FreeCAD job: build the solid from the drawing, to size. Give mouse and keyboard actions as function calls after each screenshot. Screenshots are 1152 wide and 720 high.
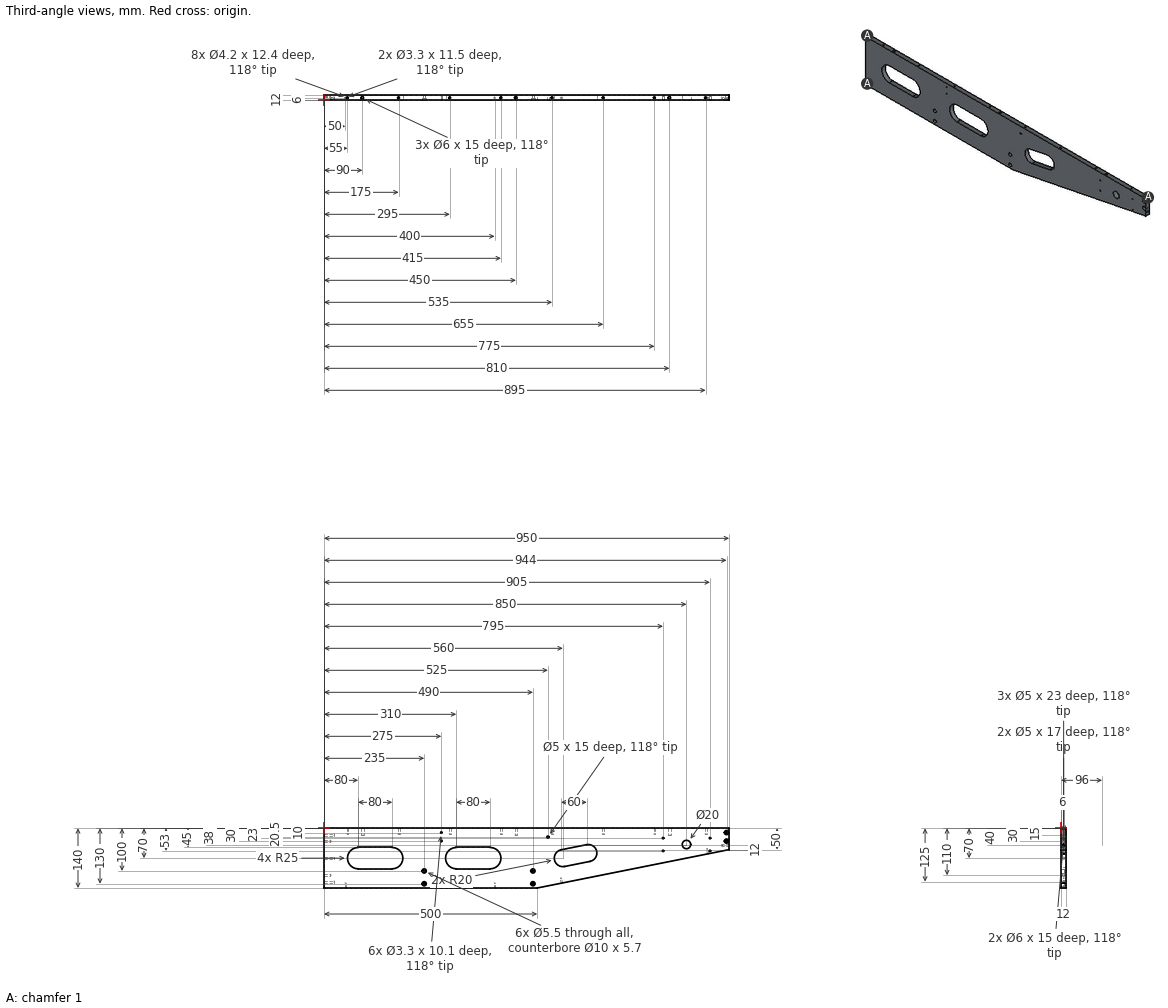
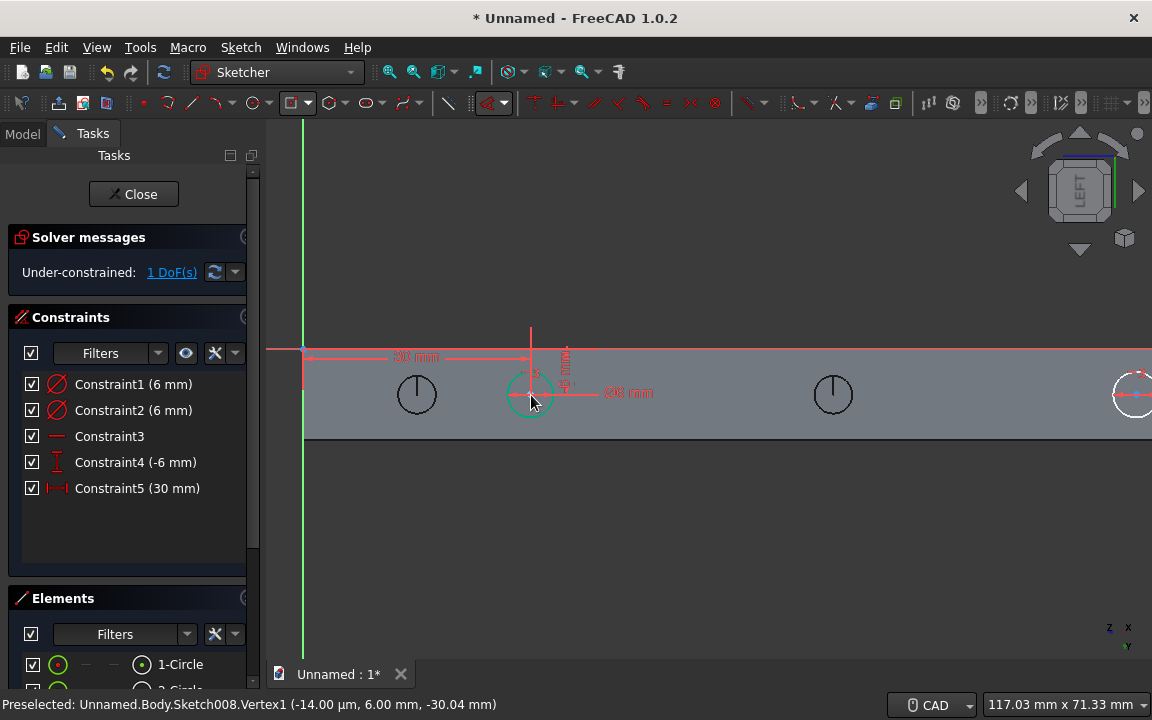
scroll(530, 396, down, 3)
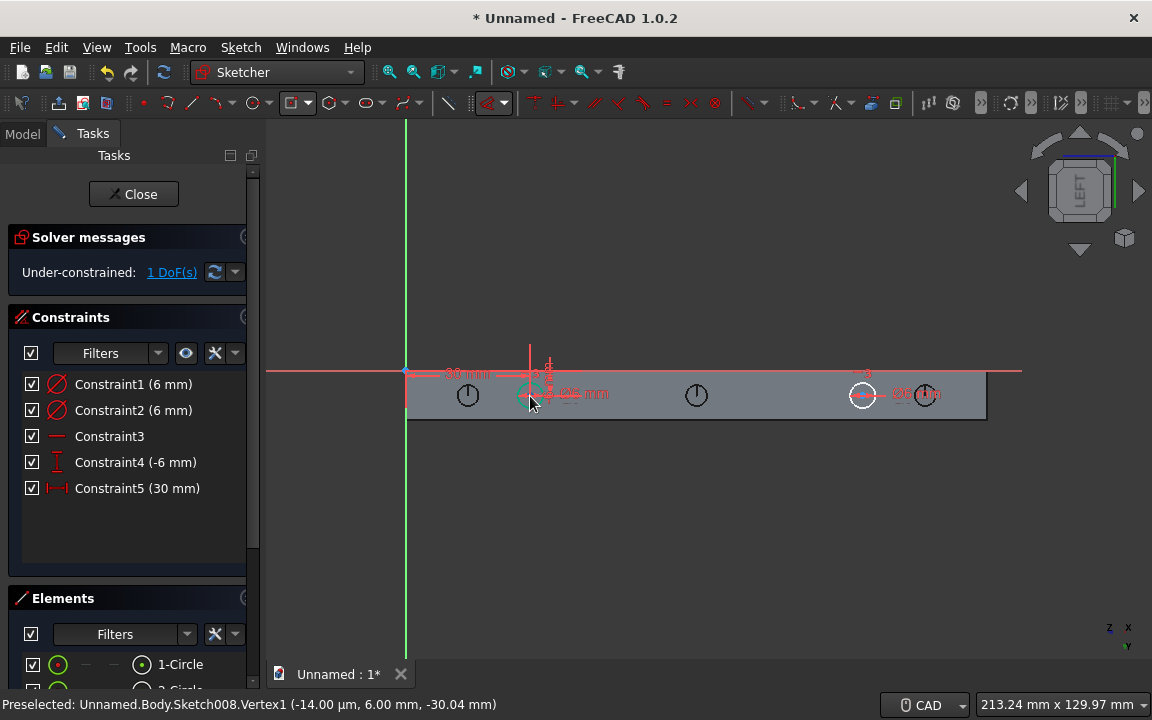
click(863, 396)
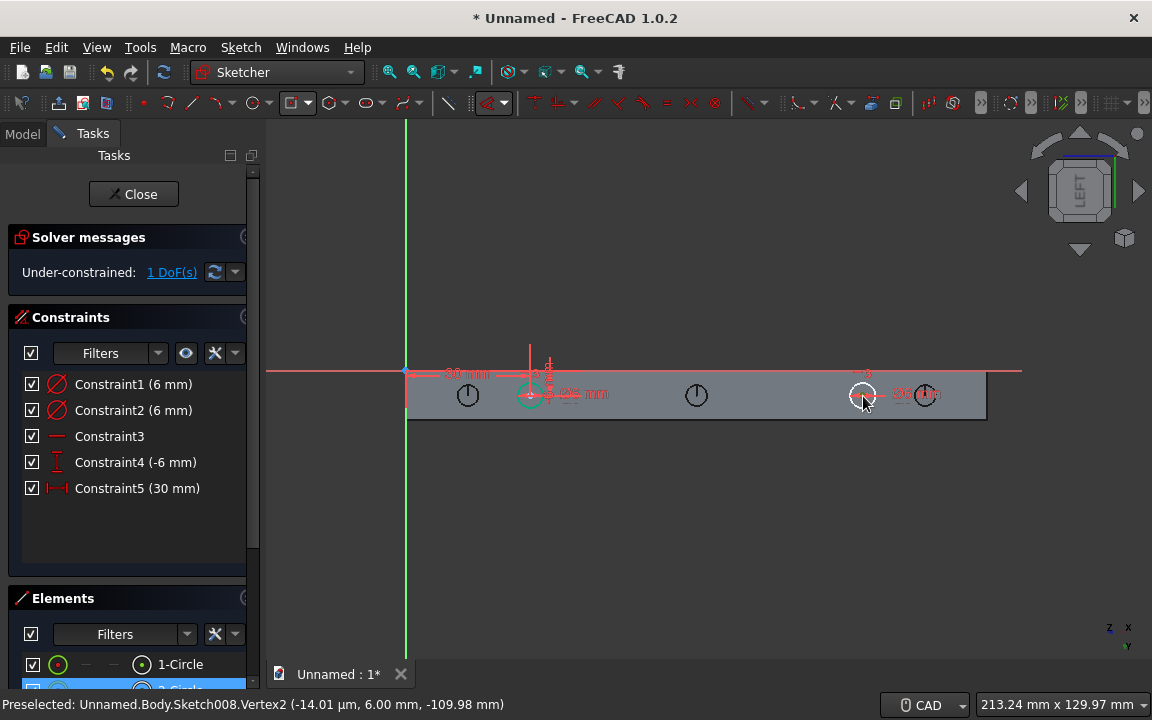
click(506, 104)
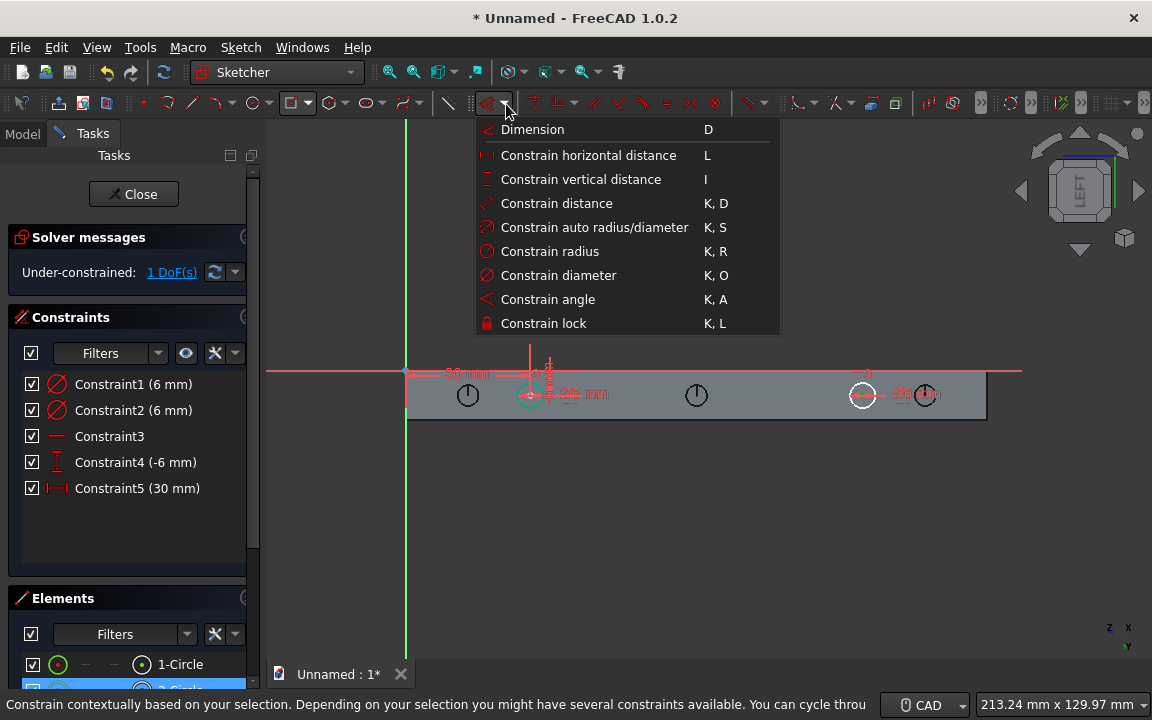
click(628, 155)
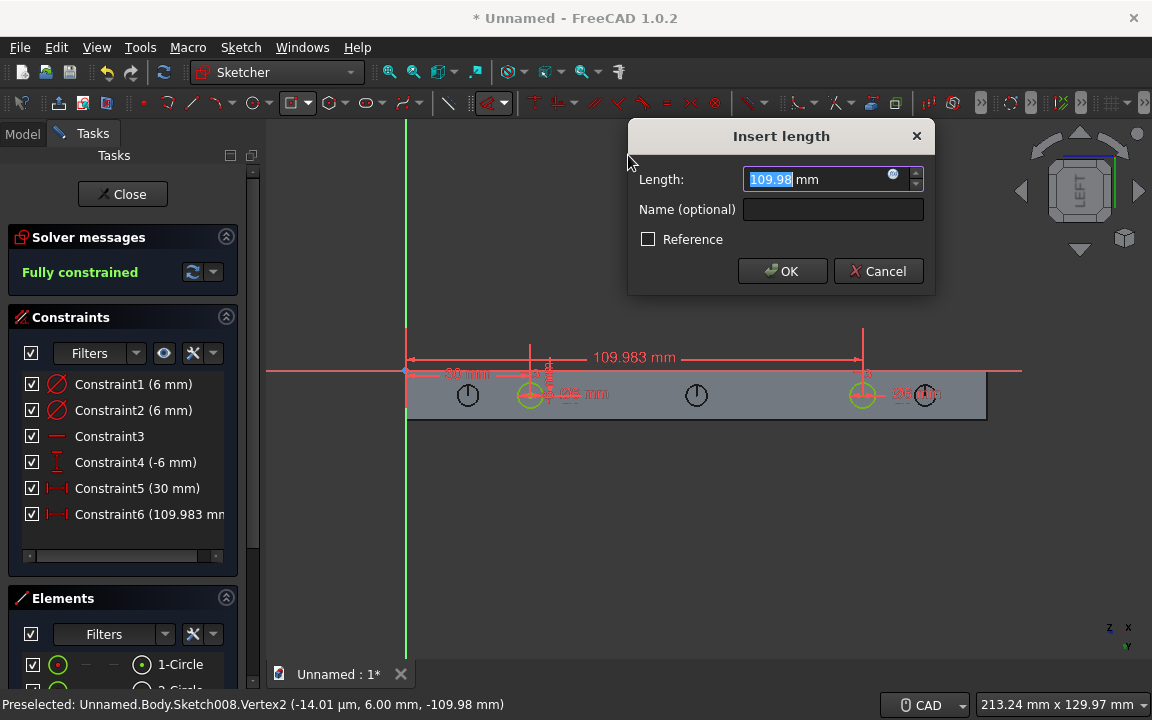
text(110)
key(Return)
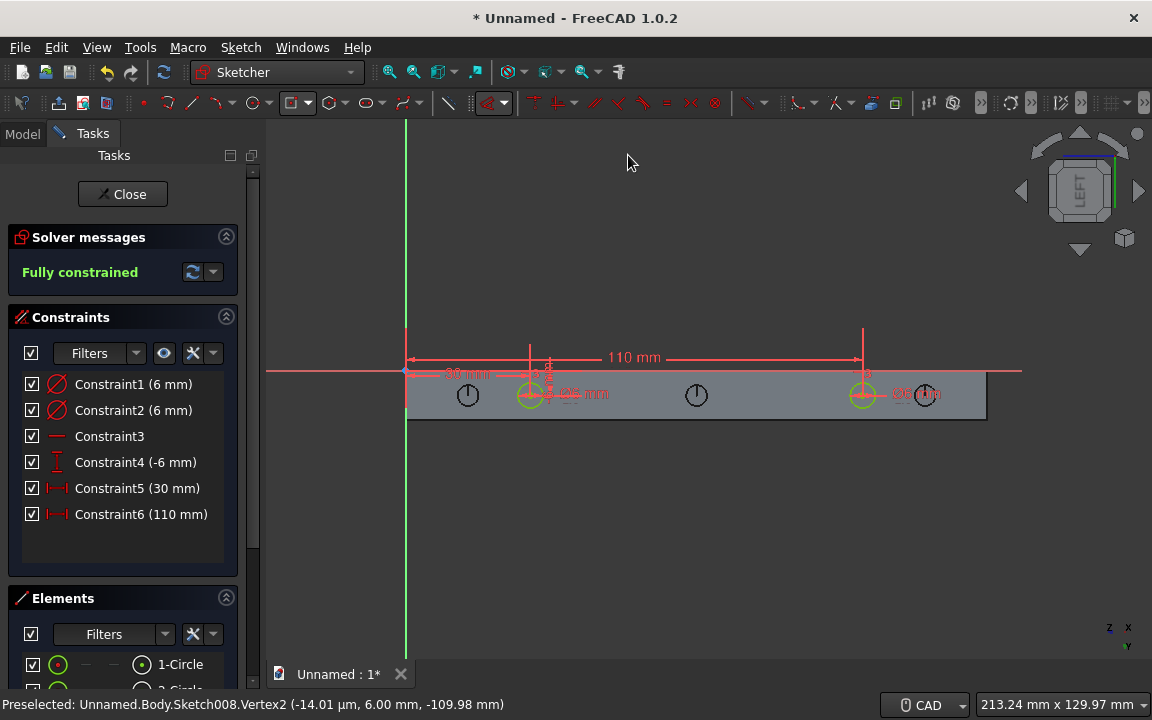
click(123, 194)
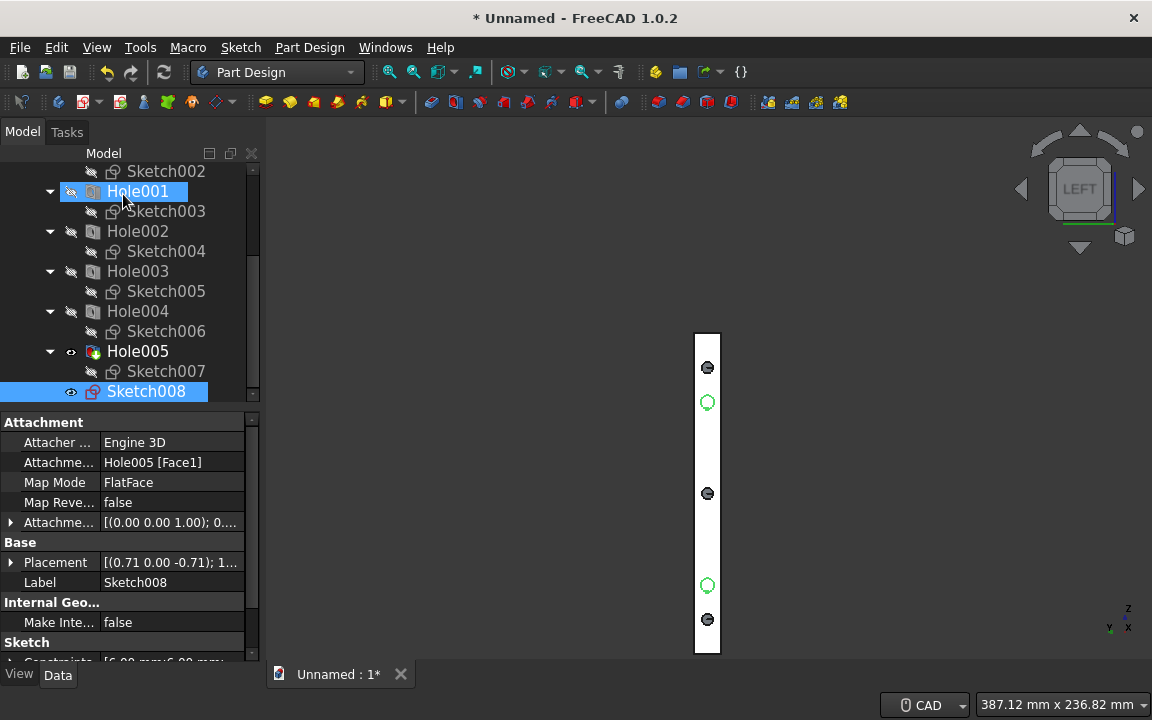
click(456, 102)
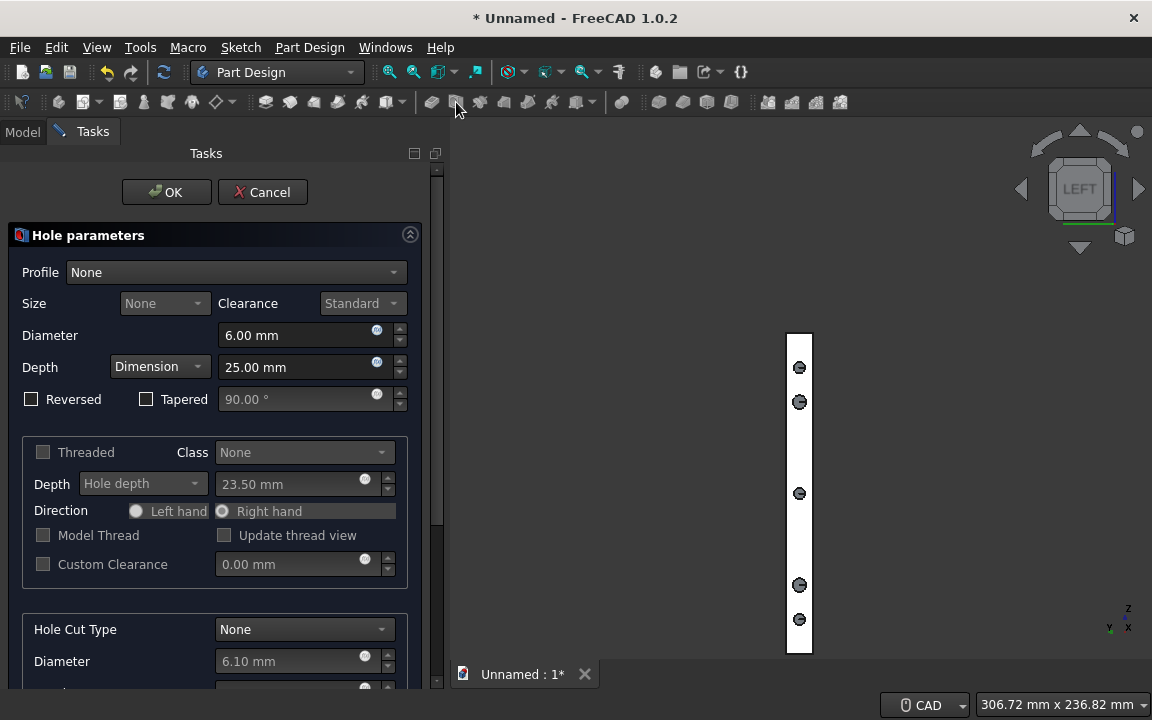
triple_click(305, 335)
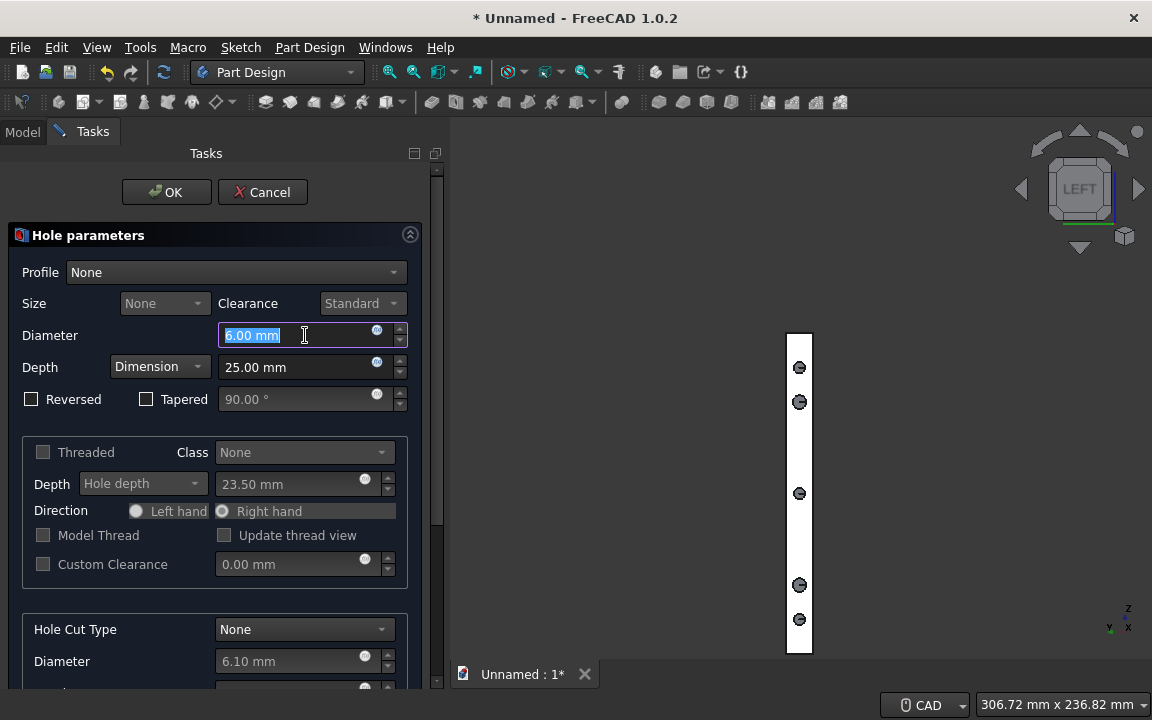
text(6)
key(Tab)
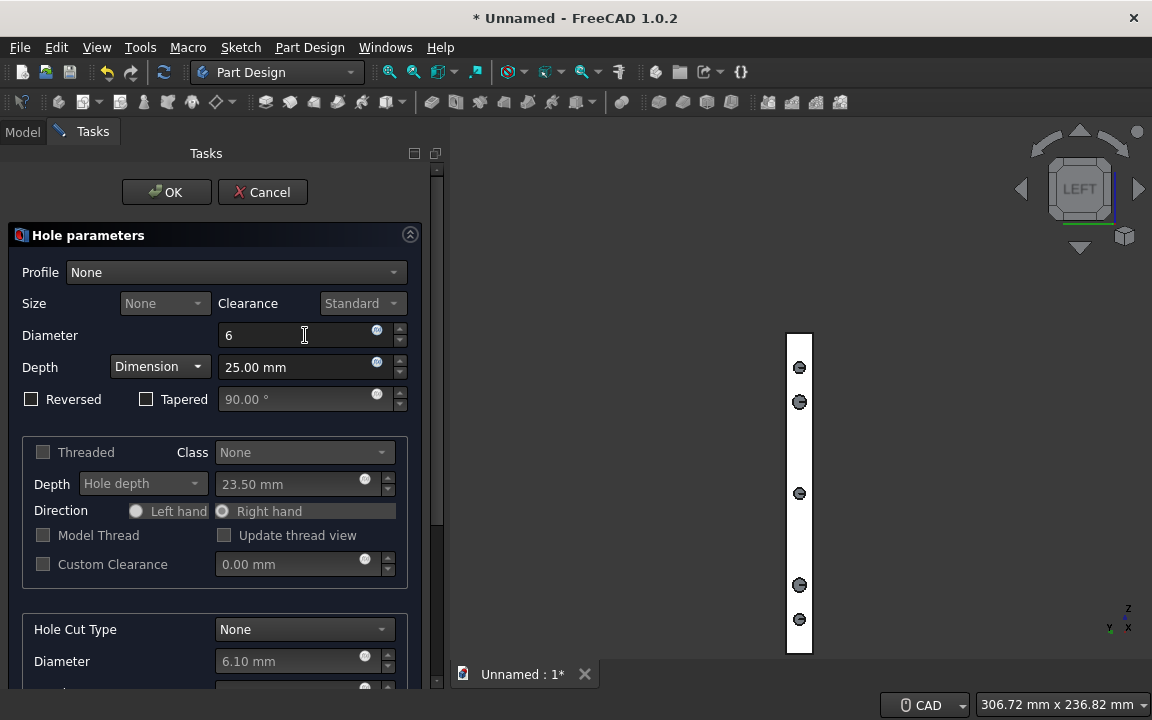
triple_click(305, 367)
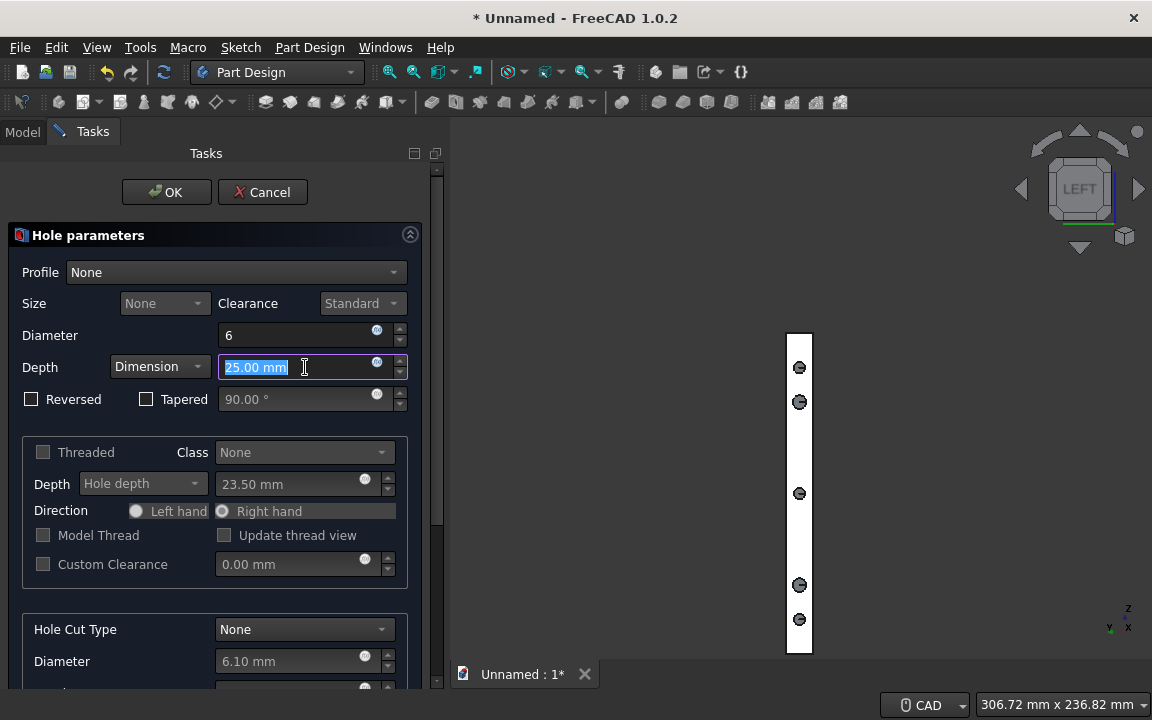
text(15)
key(Tab)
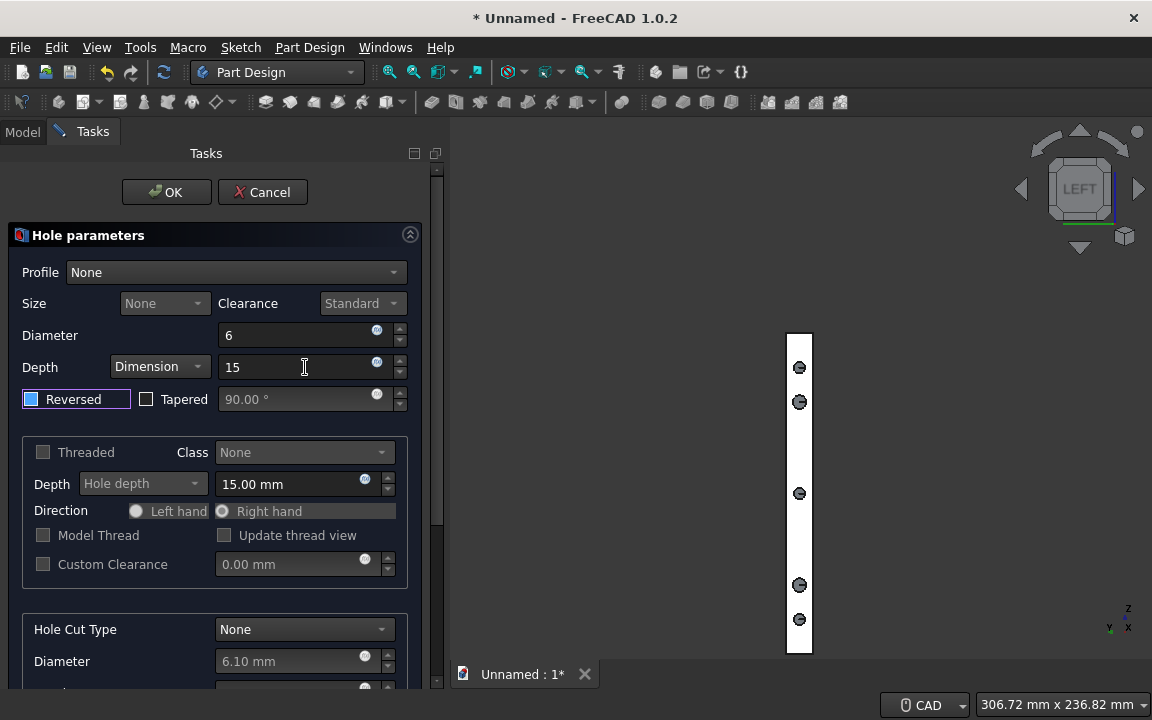
click(167, 192)